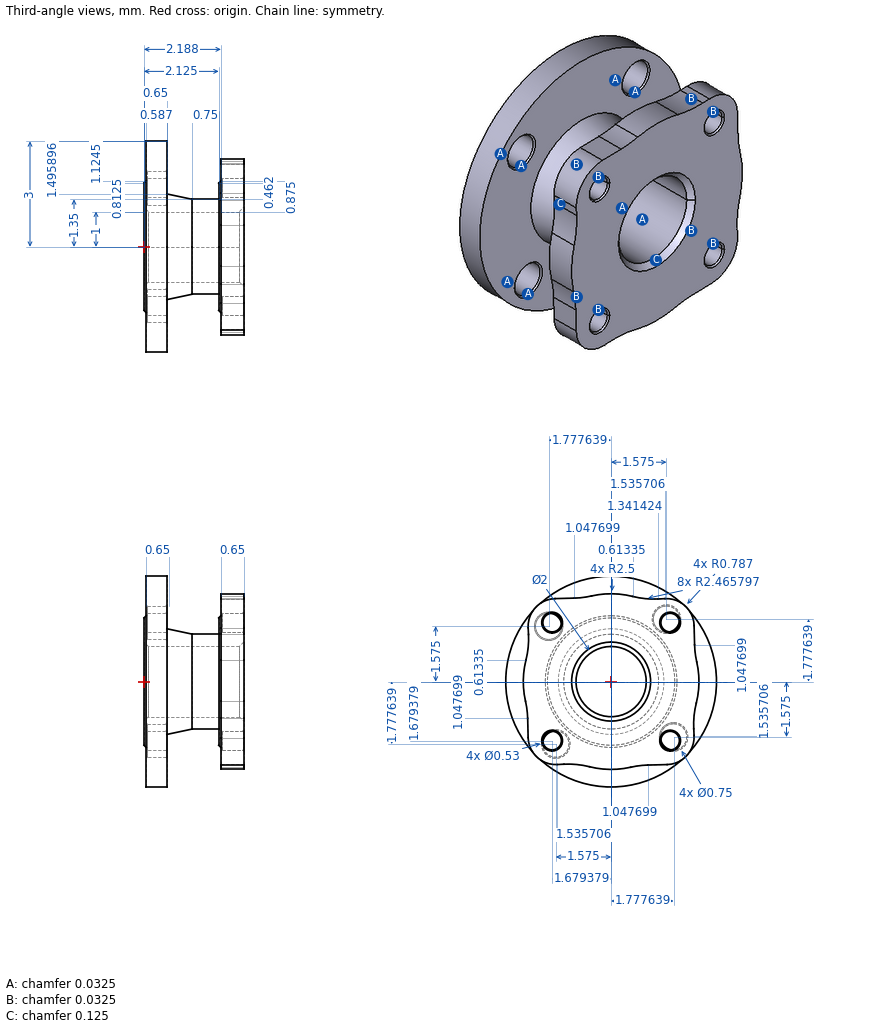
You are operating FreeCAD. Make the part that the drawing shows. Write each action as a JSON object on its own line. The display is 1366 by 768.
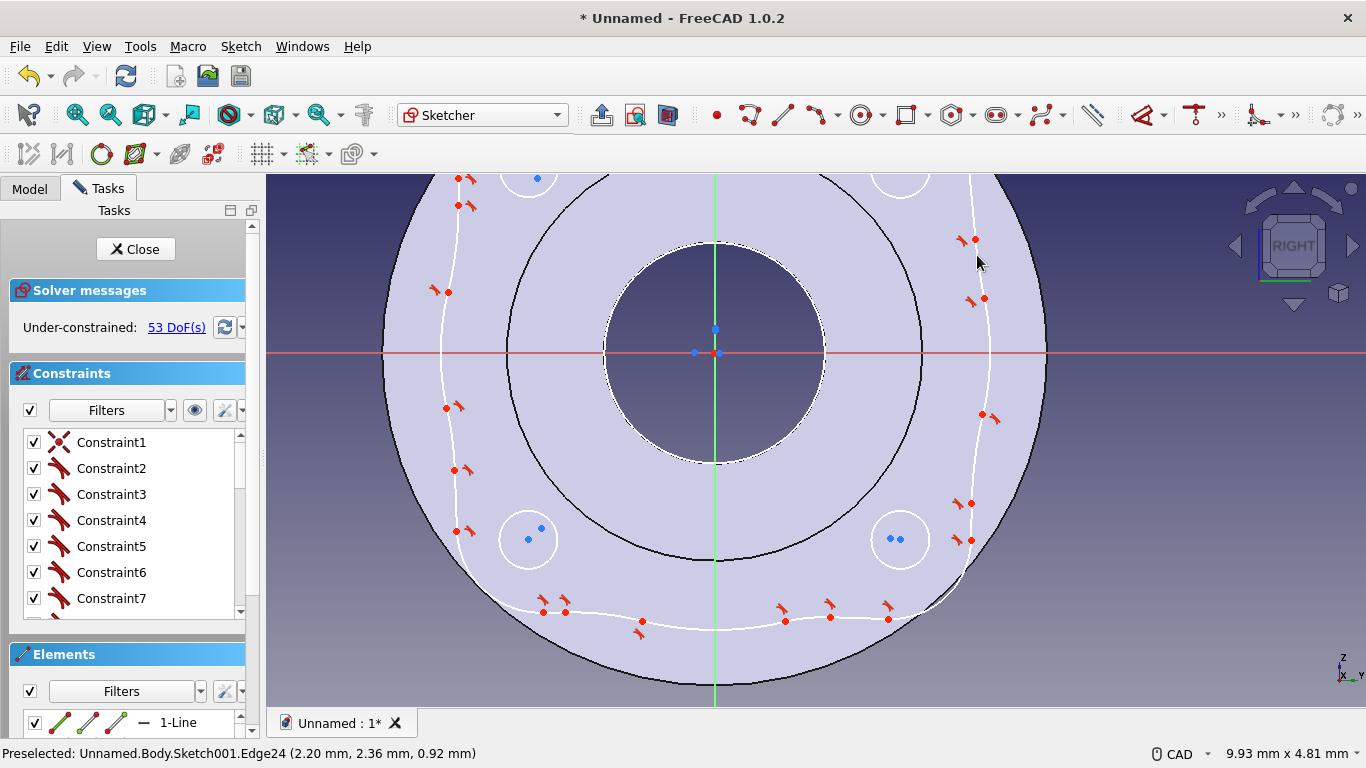
{"action": "left_click", "coordinate": [792, 275]}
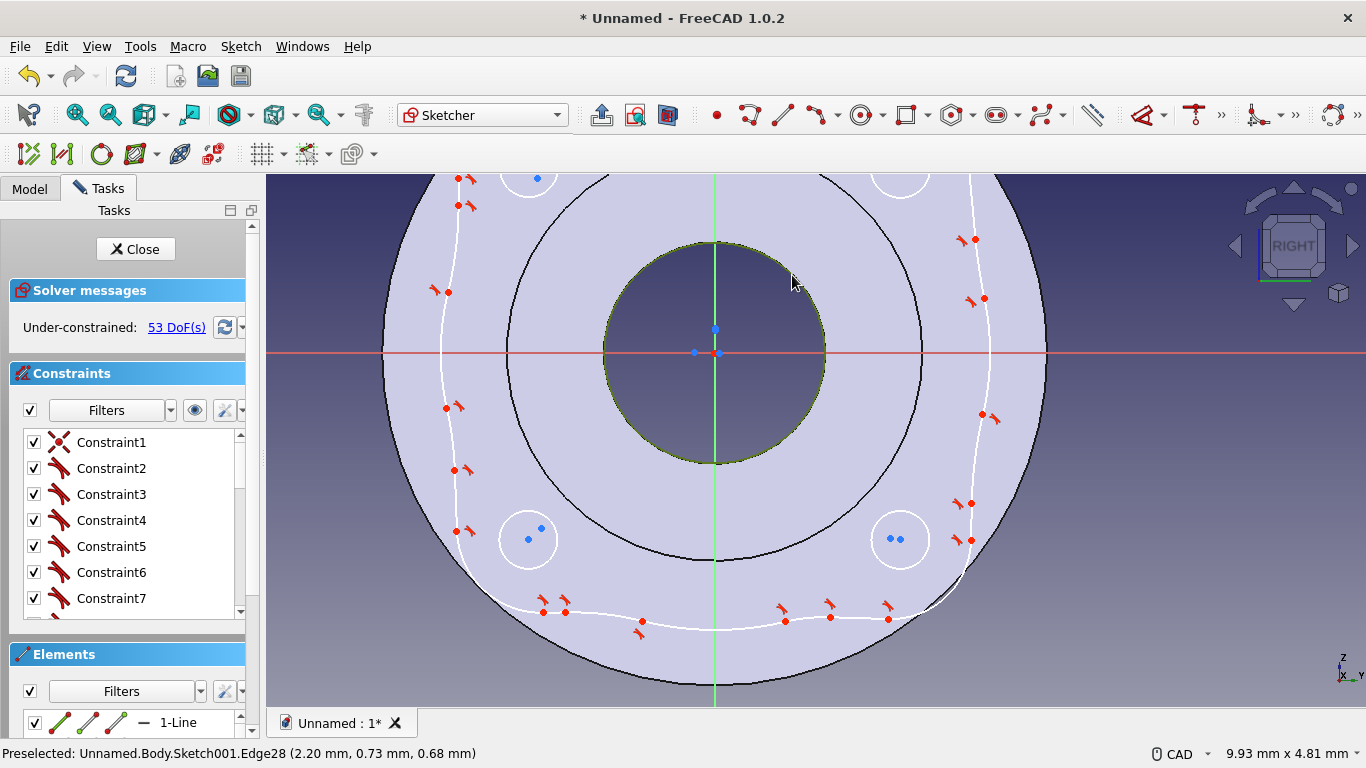
{"action": "scroll", "coordinate": [814, 618], "scroll_direction": "down", "scroll_amount": 2}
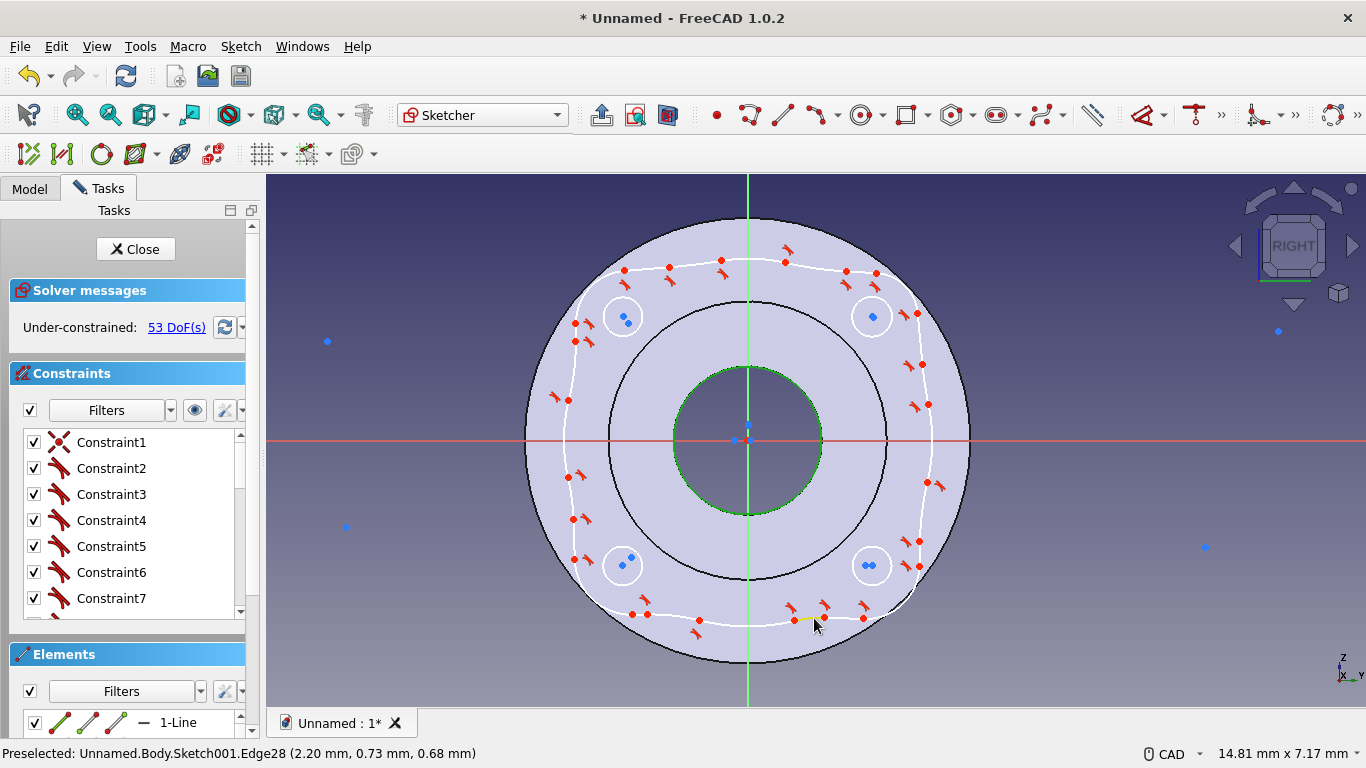
{"action": "left_click", "coordinate": [767, 260]}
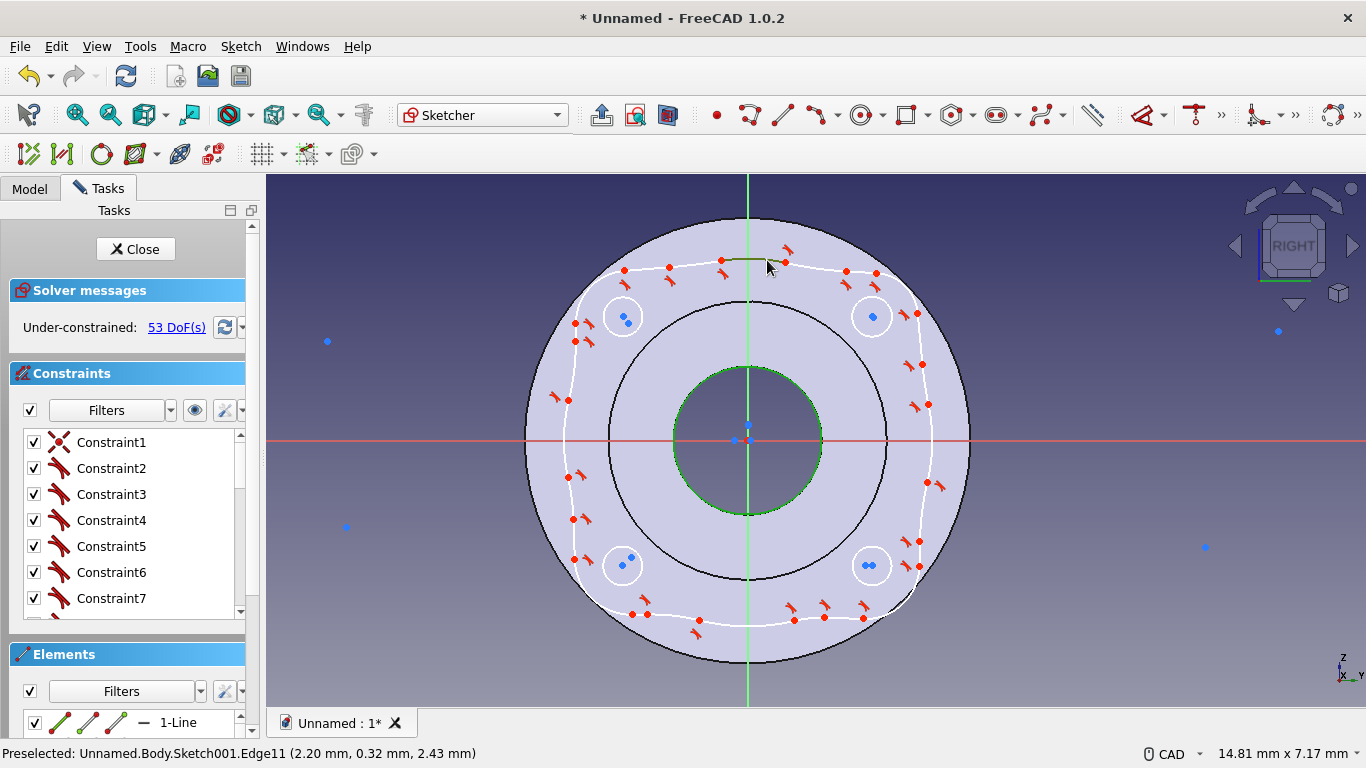
{"action": "left_click", "coordinate": [1194, 116]}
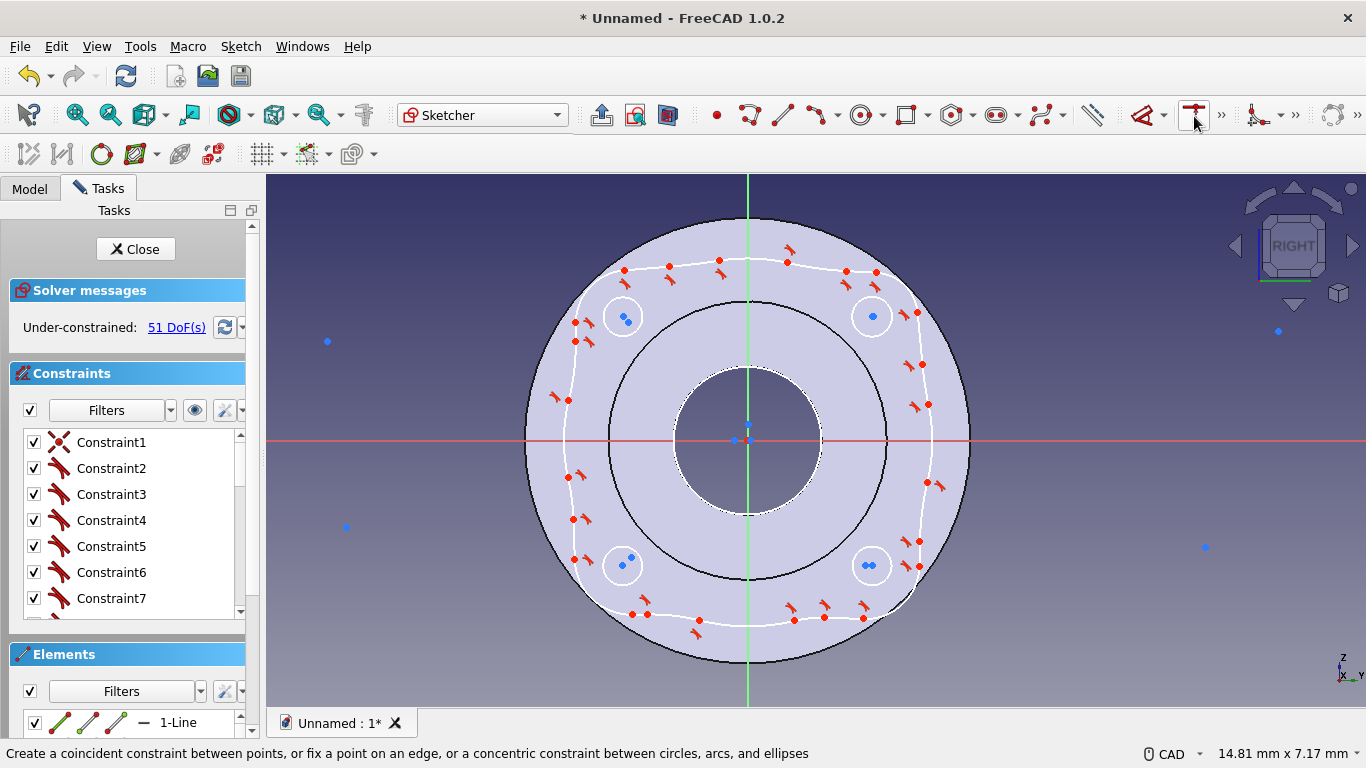
{"action": "left_click", "coordinate": [800, 388]}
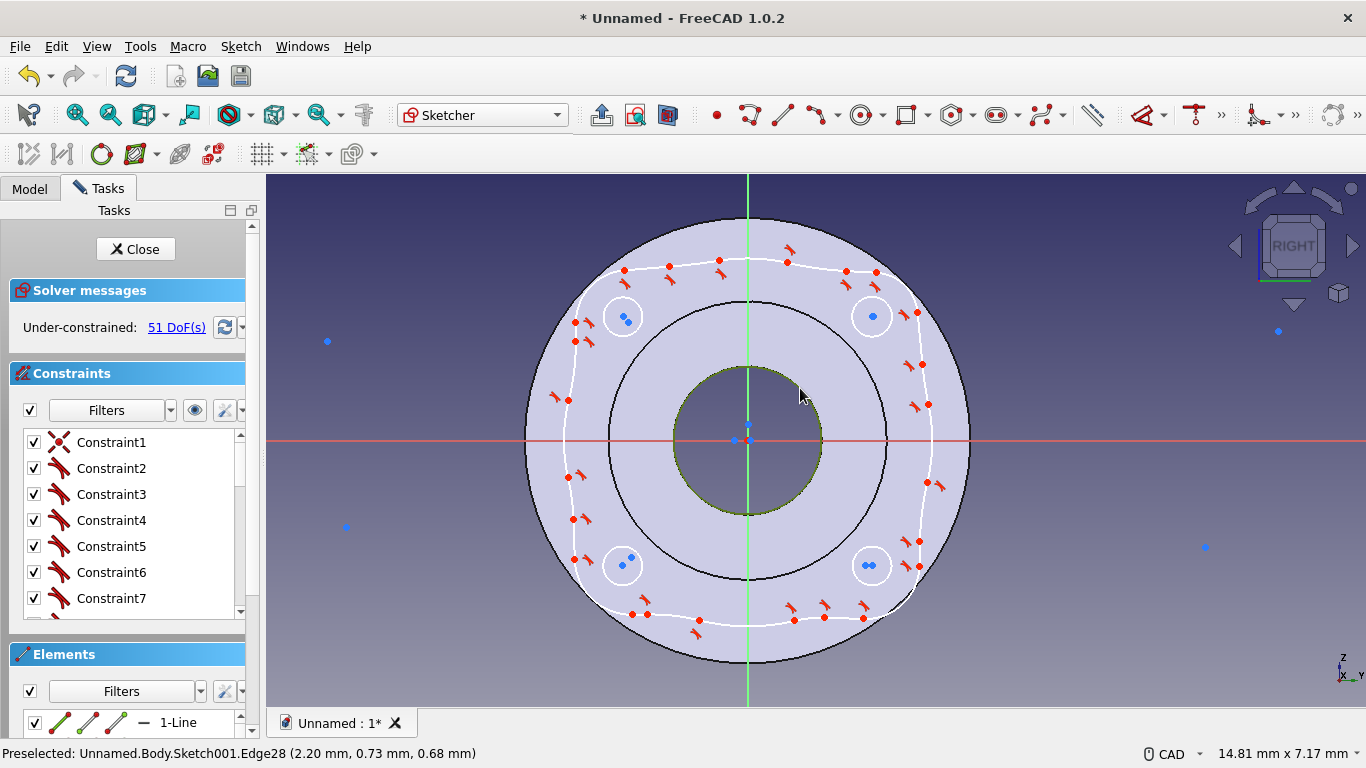
{"action": "left_click", "coordinate": [565, 423]}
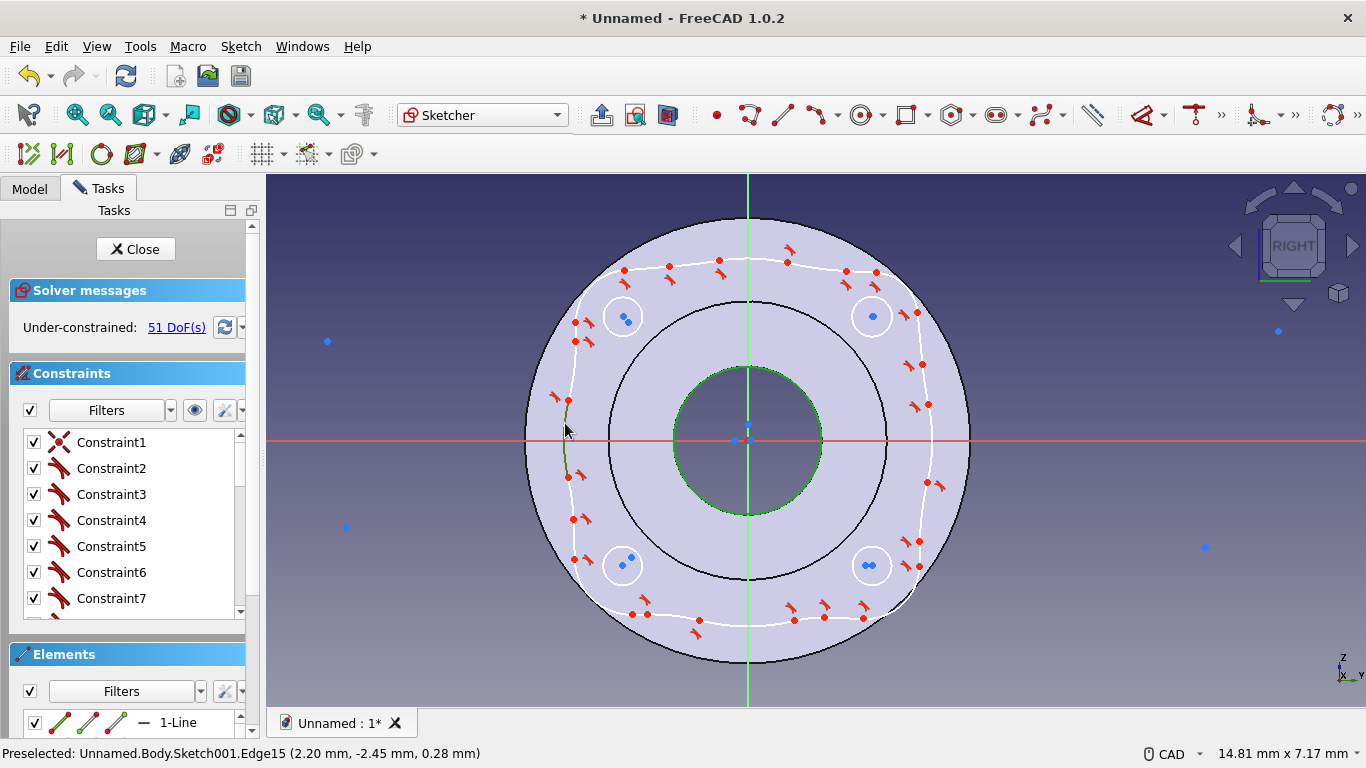
{"action": "left_click", "coordinate": [1194, 116]}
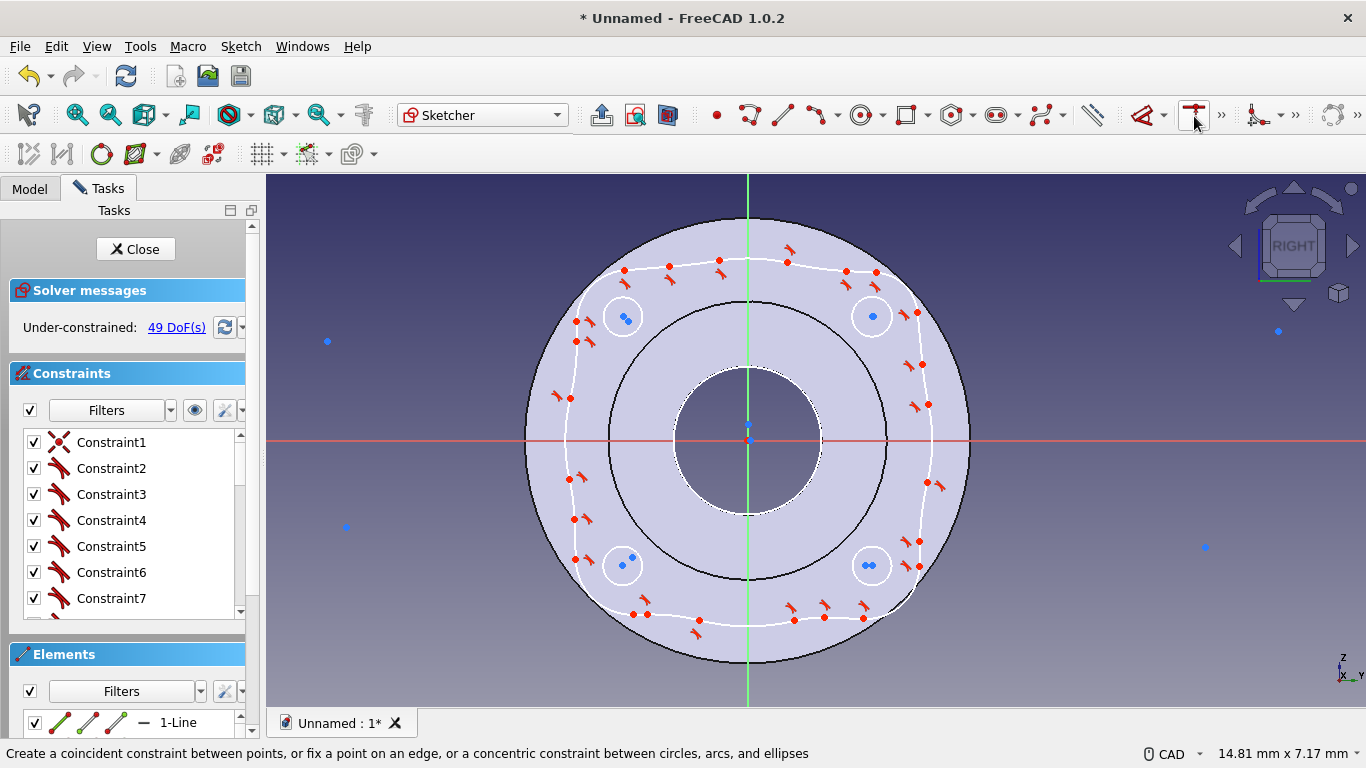
{"action": "left_click", "coordinate": [800, 388]}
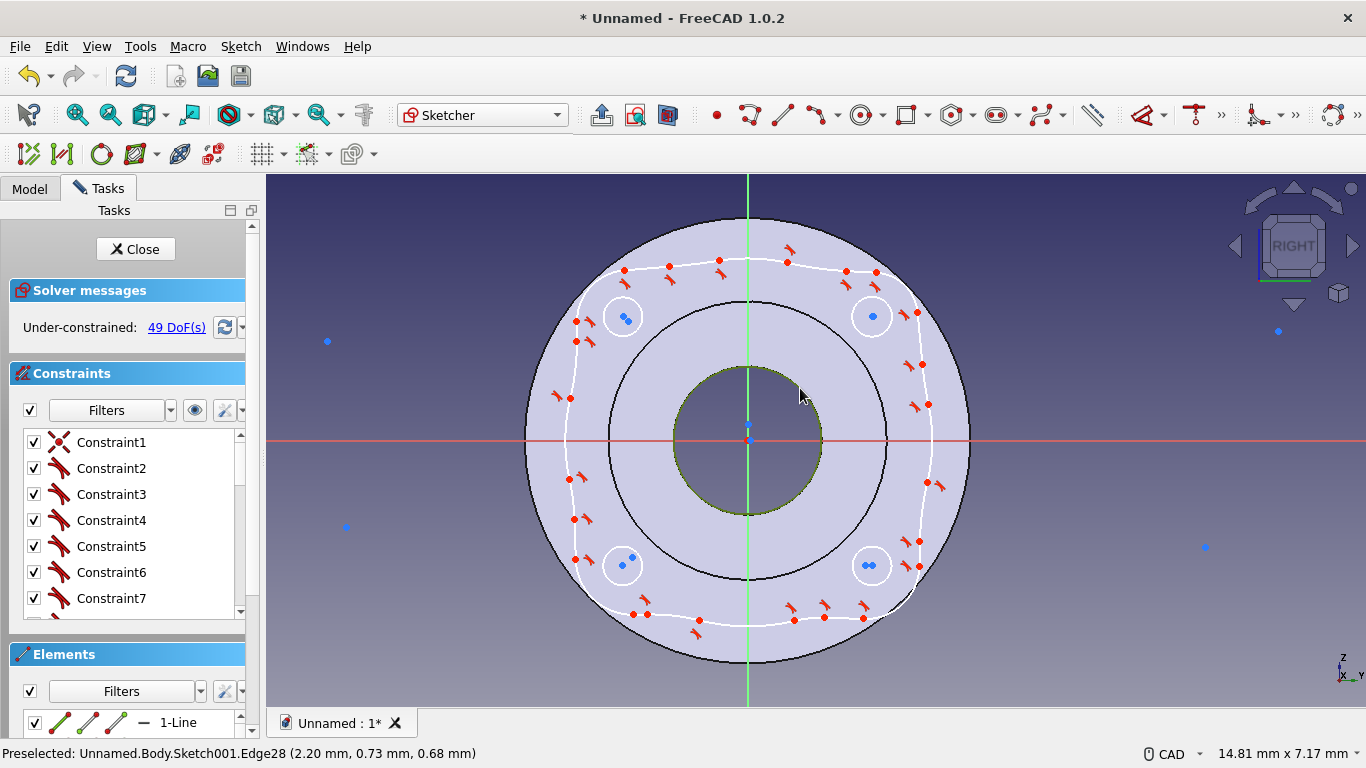
{"action": "left_click", "coordinate": [728, 625]}